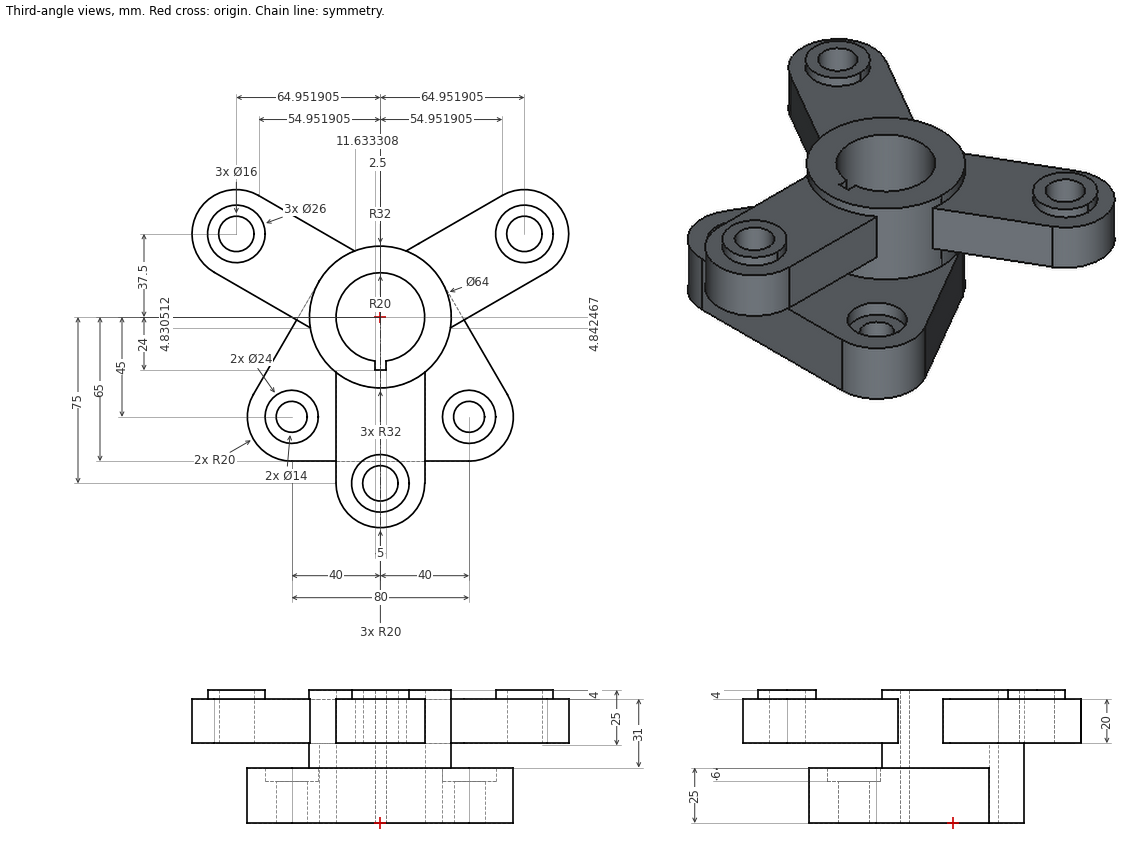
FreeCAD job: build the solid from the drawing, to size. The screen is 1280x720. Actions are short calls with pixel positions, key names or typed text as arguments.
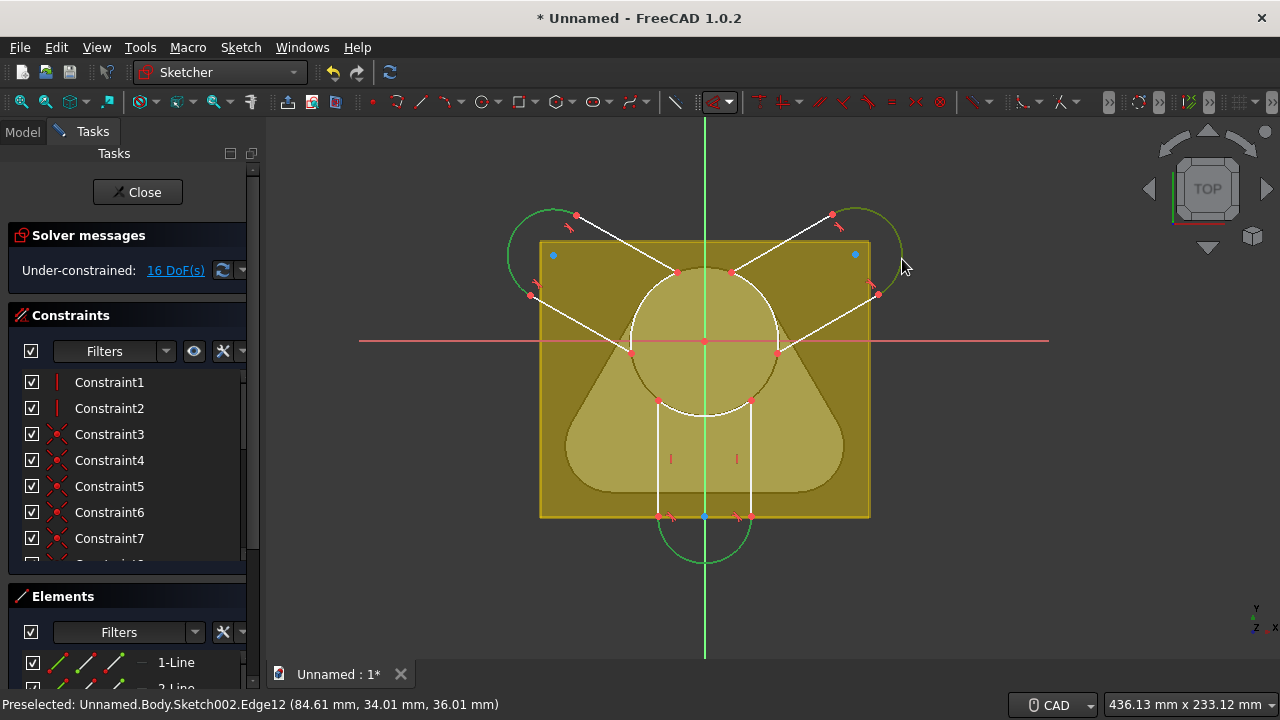
key(e)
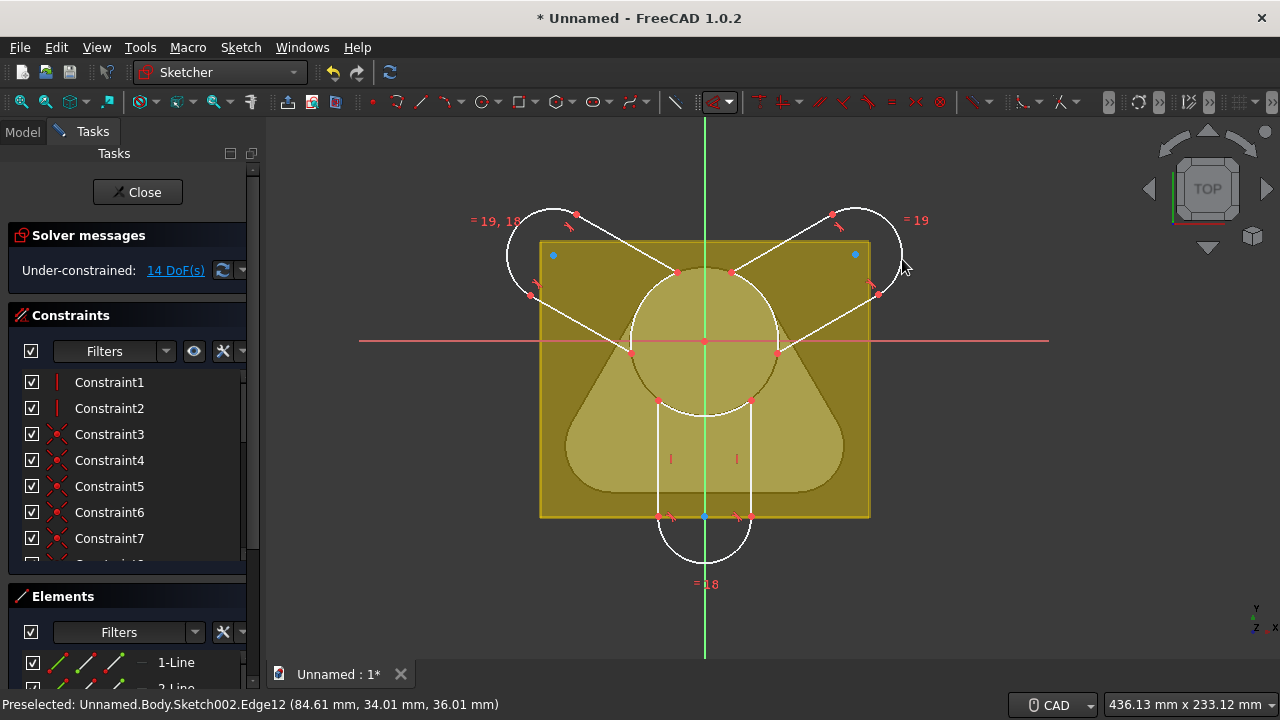
click(685, 414)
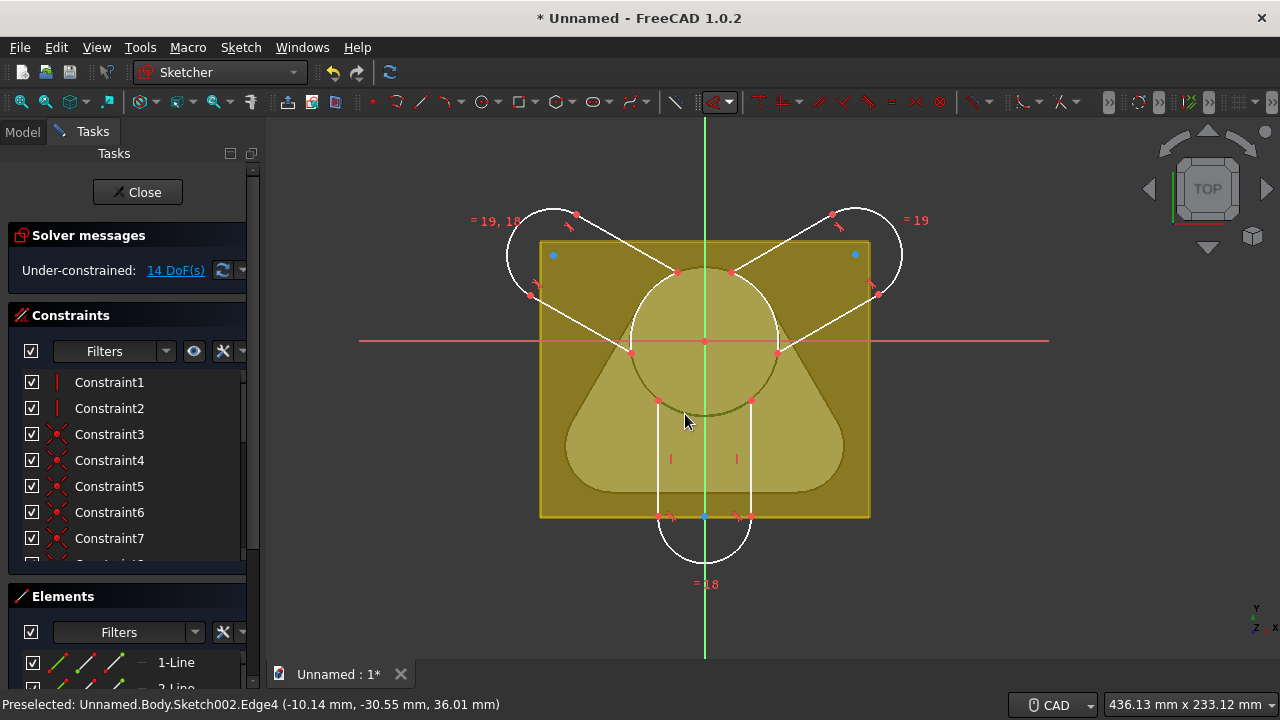
click(653, 289)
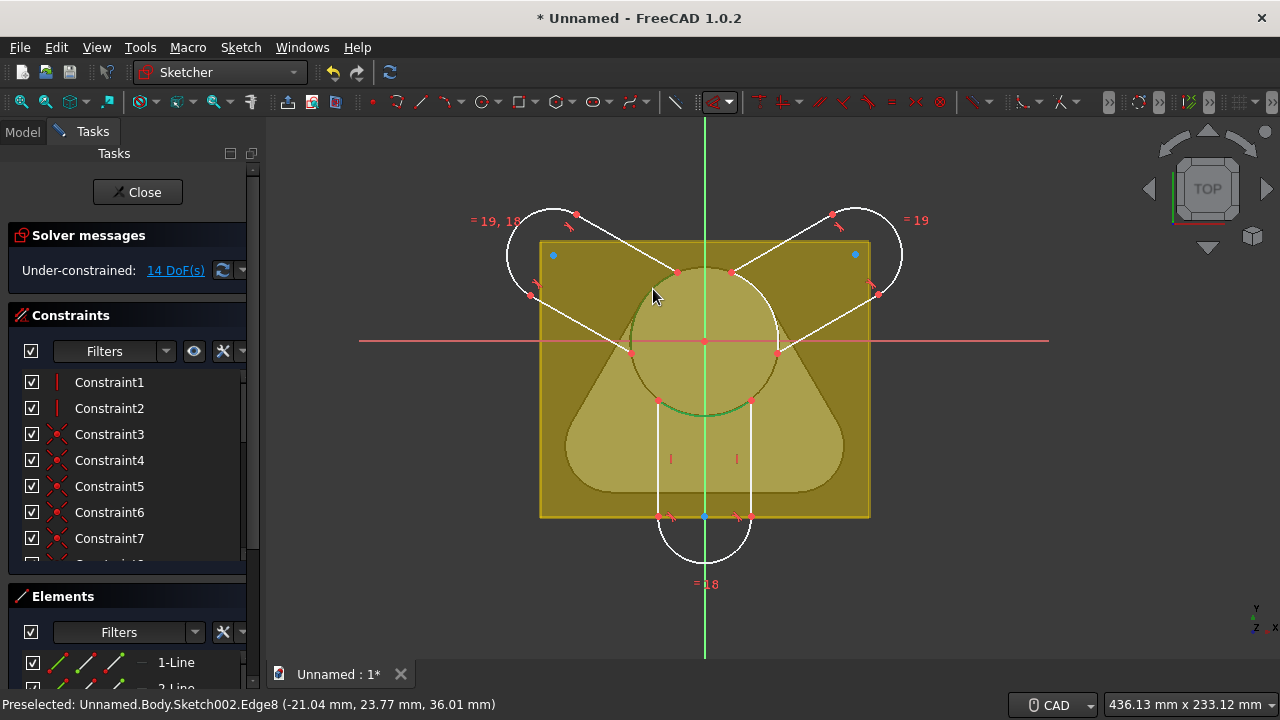
click(776, 323)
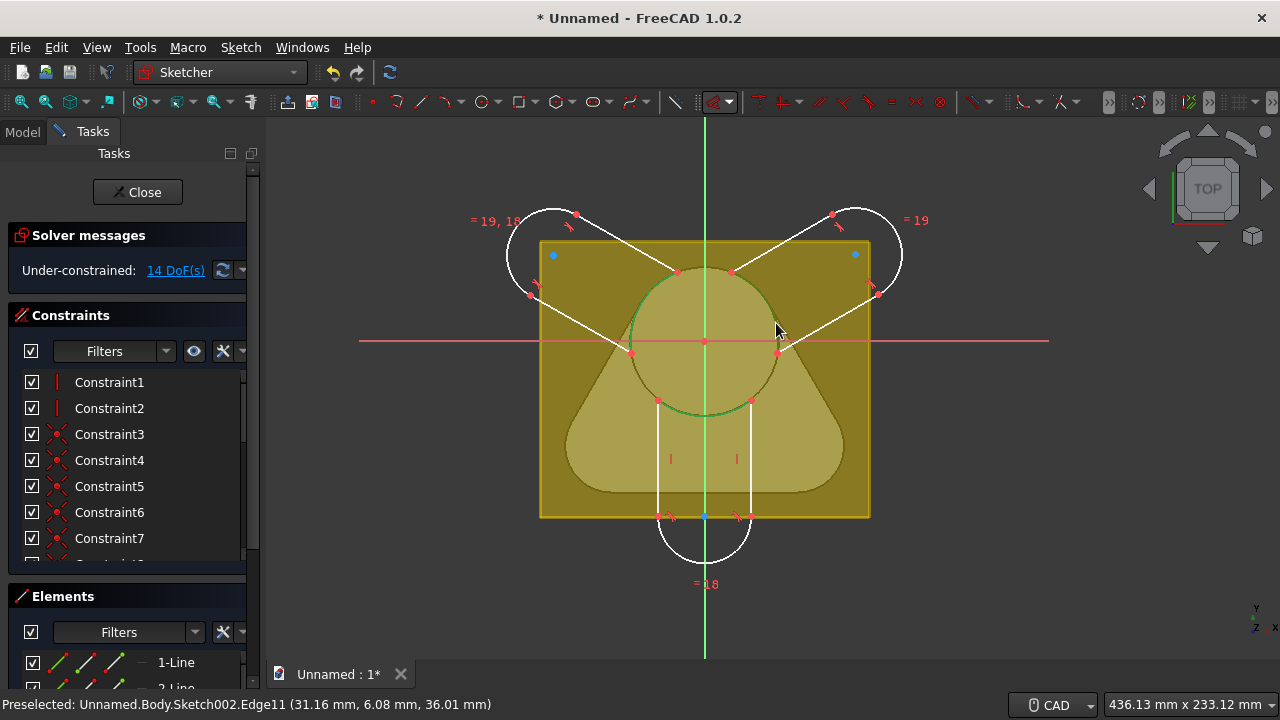
click(892, 102)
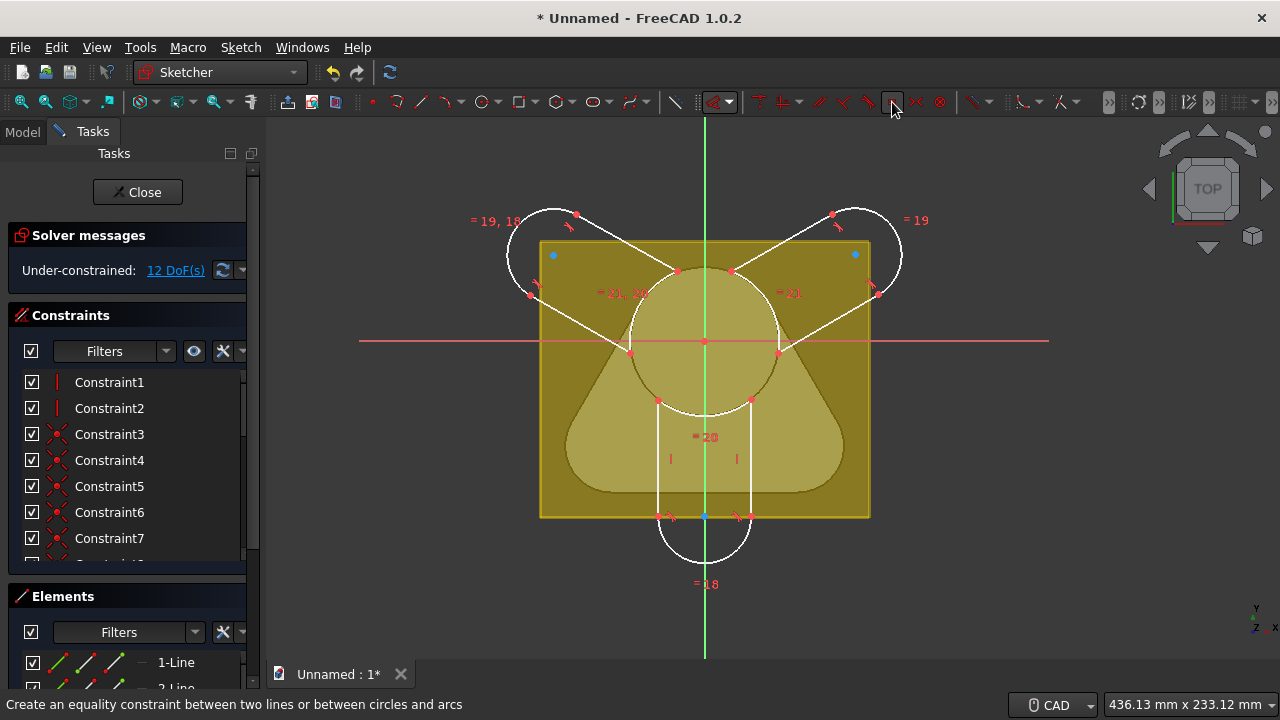
click(705, 517)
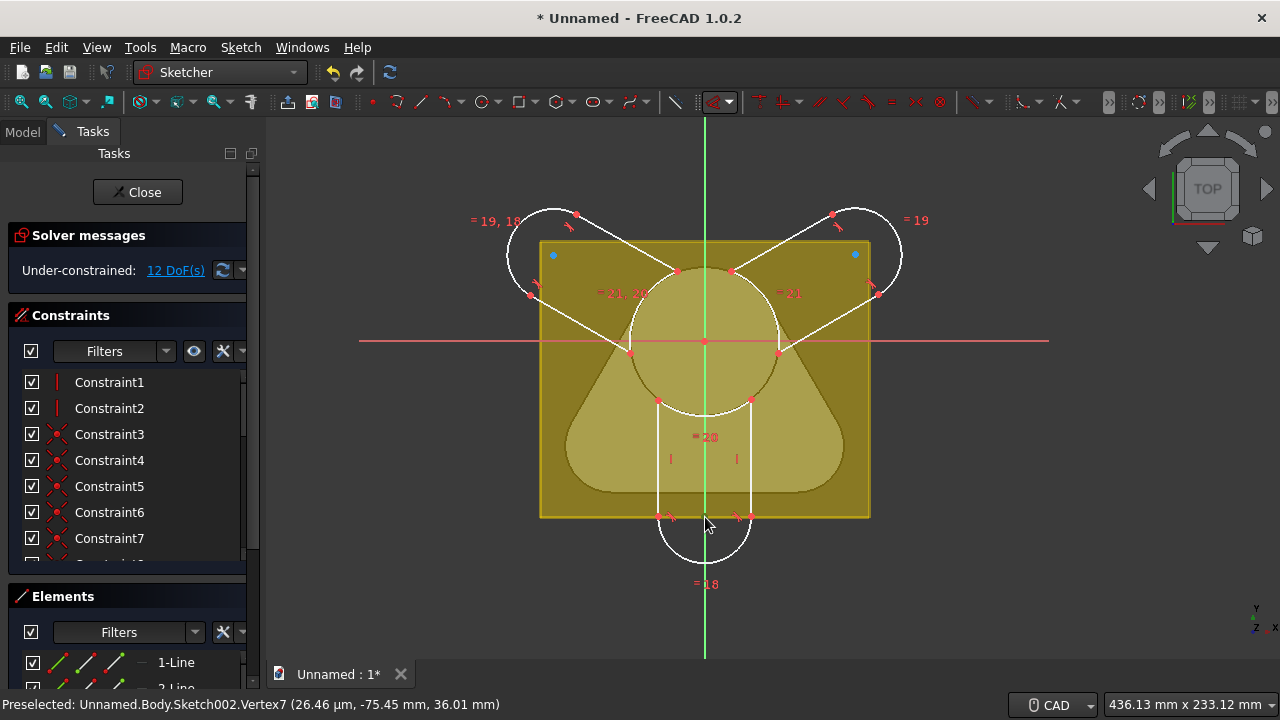
click(705, 596)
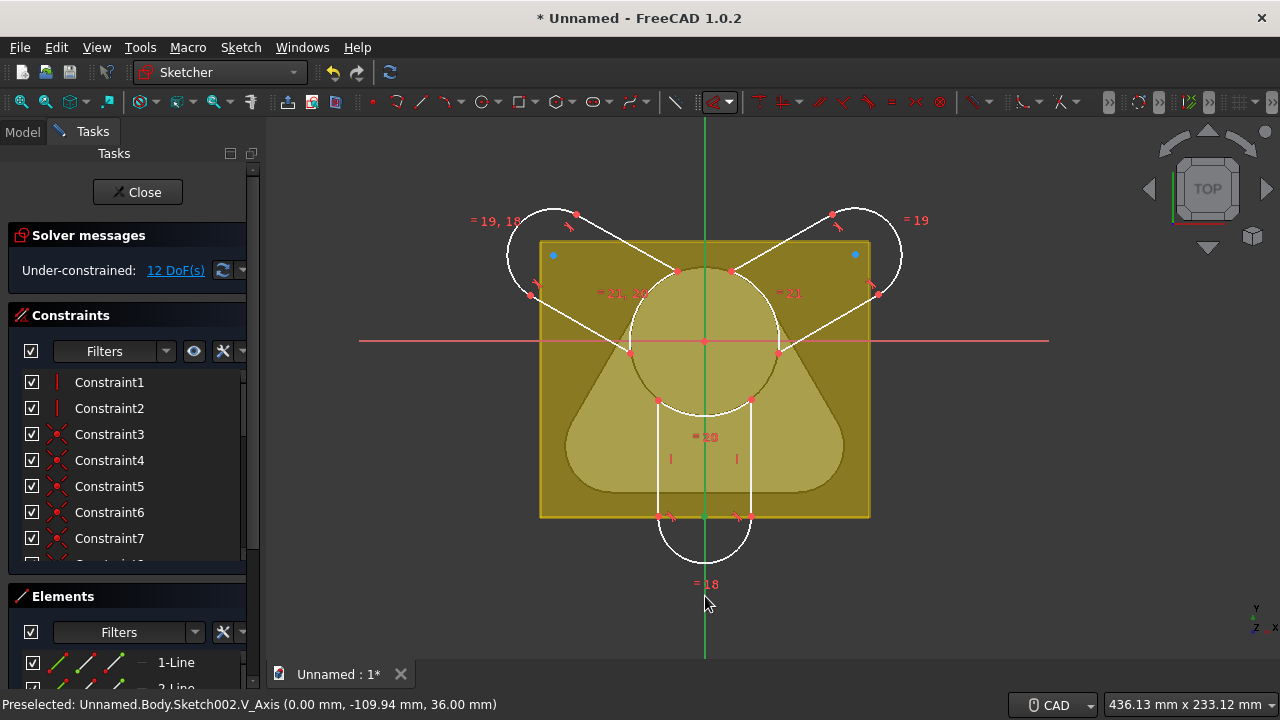
key(c)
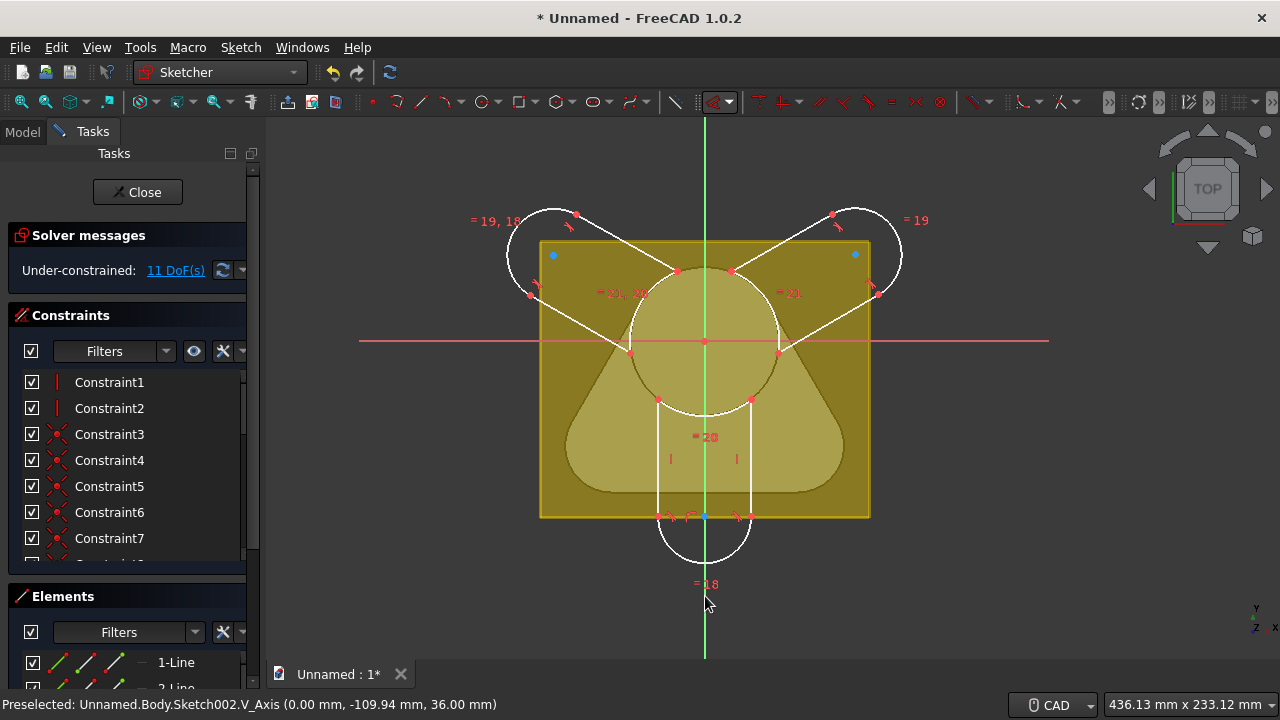
click(554, 255)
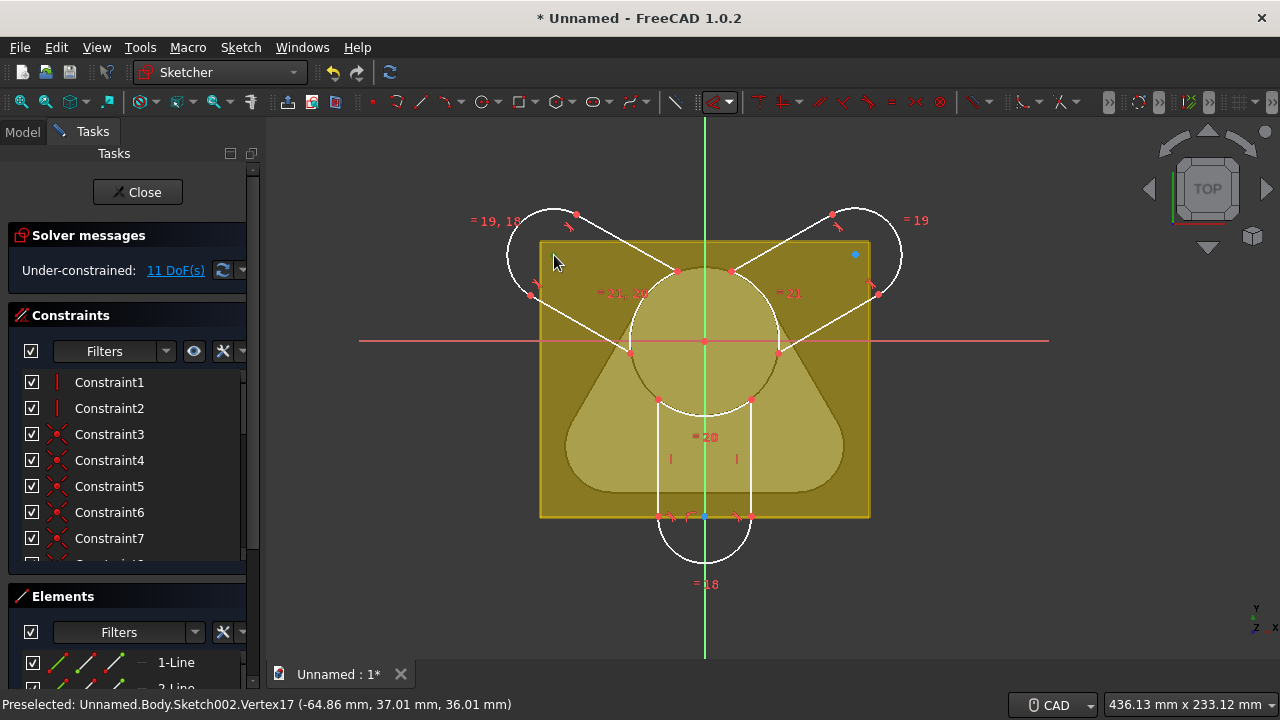
click(855, 255)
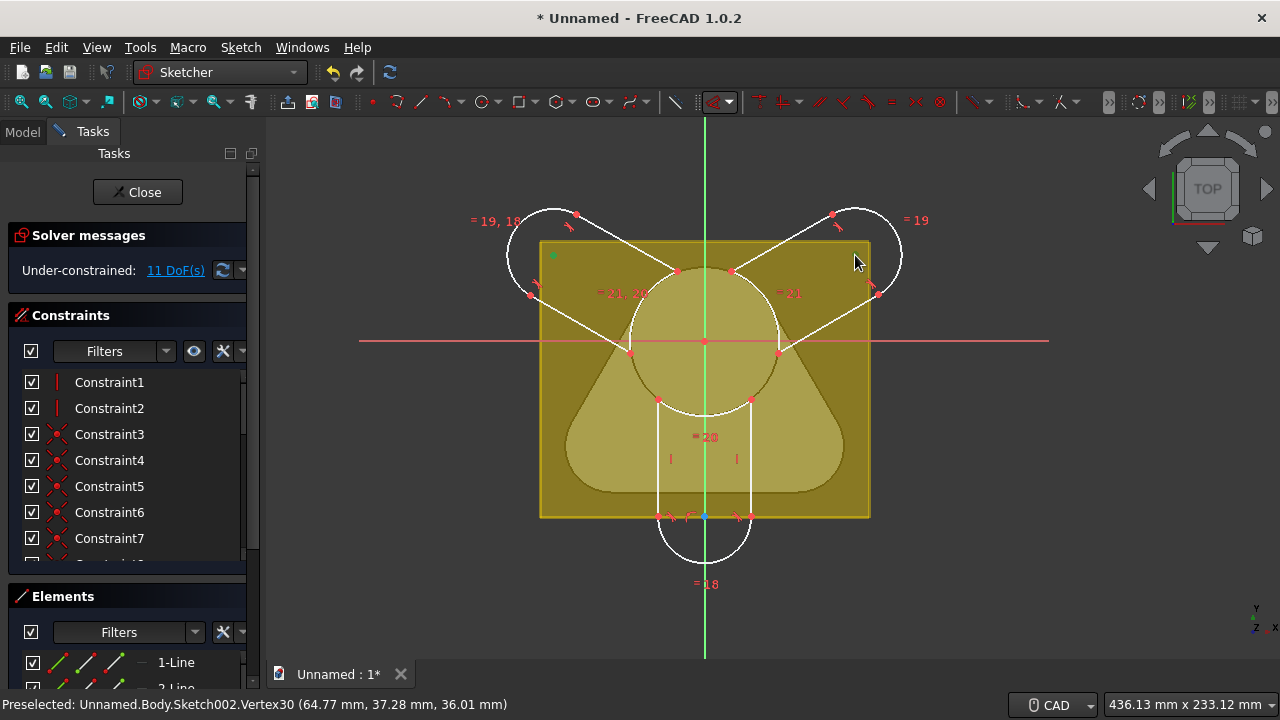
click(705, 596)